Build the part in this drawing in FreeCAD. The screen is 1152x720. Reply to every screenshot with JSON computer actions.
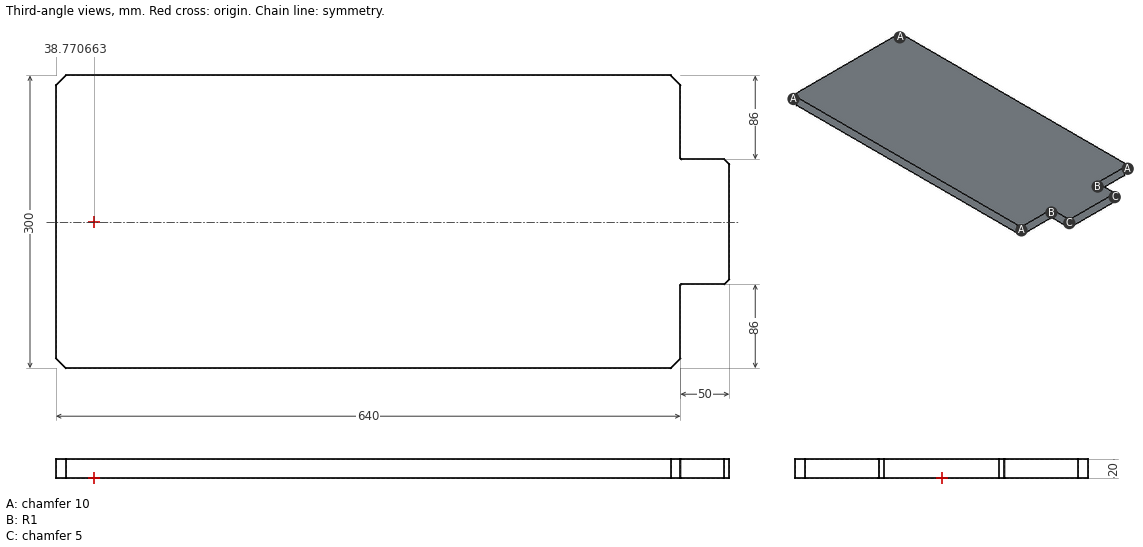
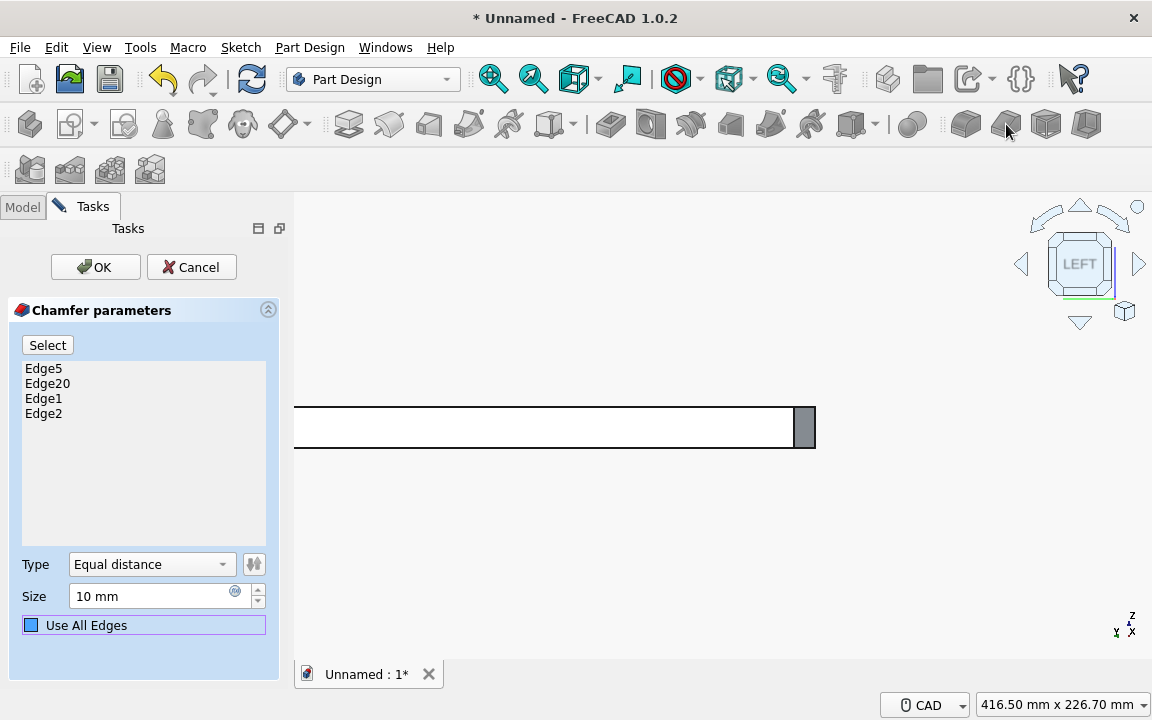
{"action": "left_click", "coordinate": [96, 267]}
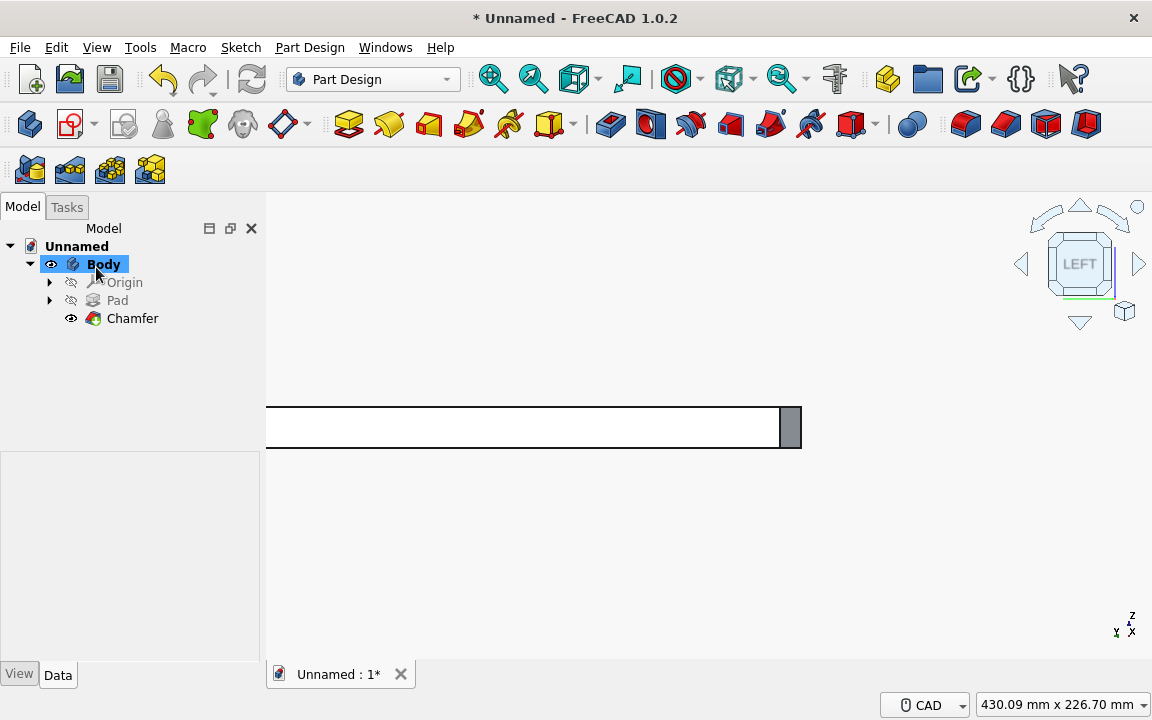
{"action": "left_click", "coordinate": [494, 80]}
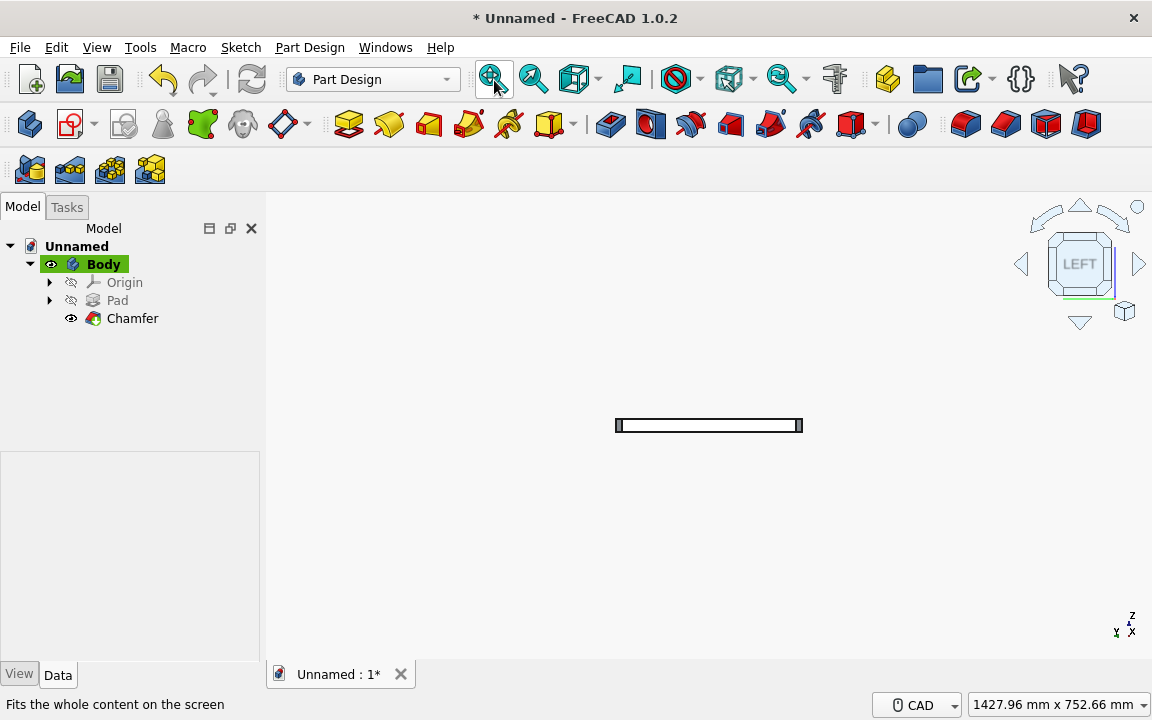
{"action": "scroll", "coordinate": [669, 424], "scroll_direction": "up", "scroll_amount": 6}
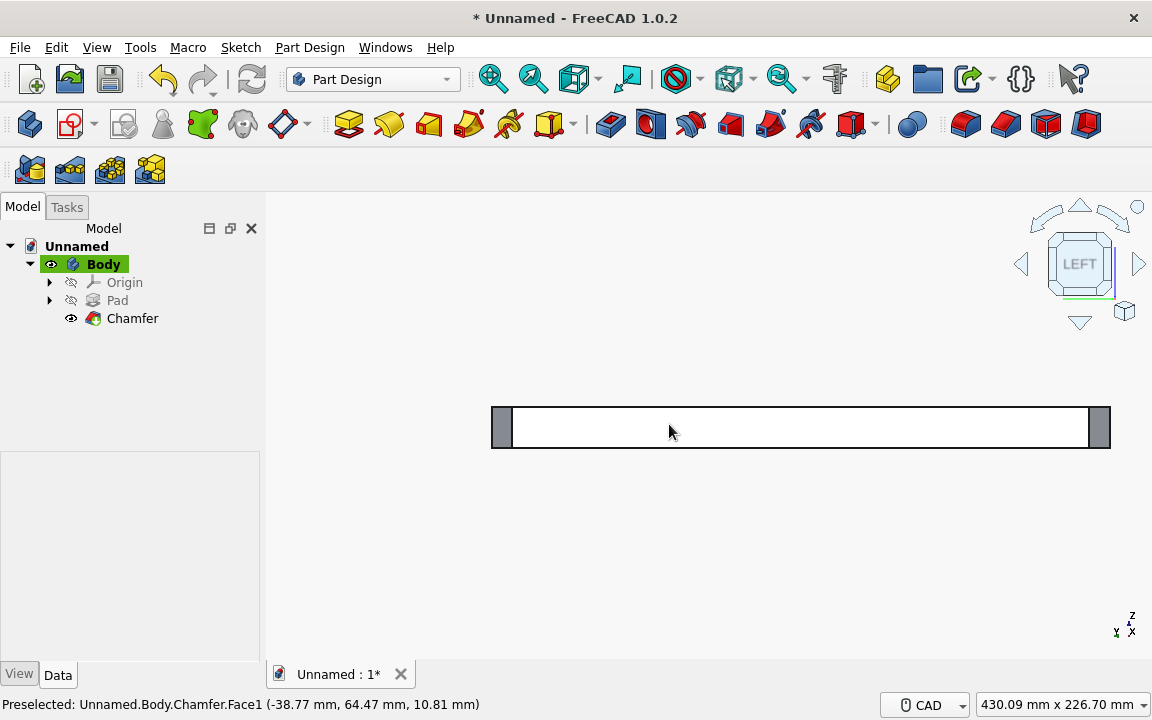
{"action": "key", "text": "v f"}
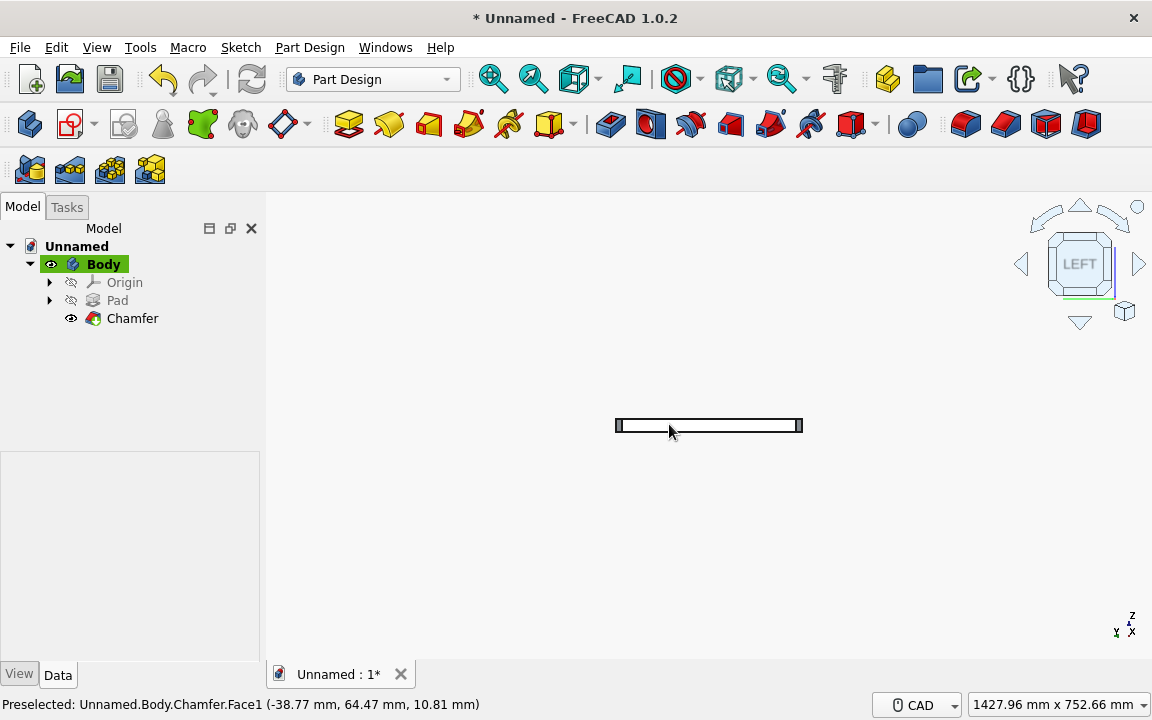
{"action": "key", "text": "0"}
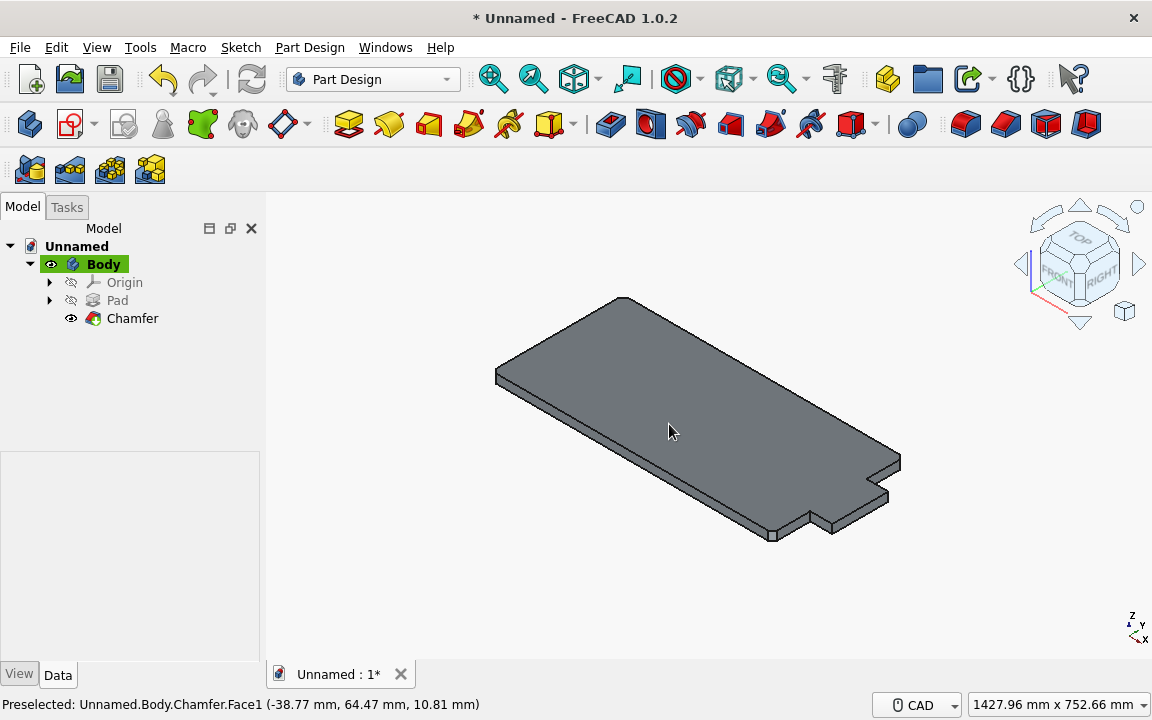
{"action": "scroll", "coordinate": [867, 483], "scroll_direction": "up", "scroll_amount": 6}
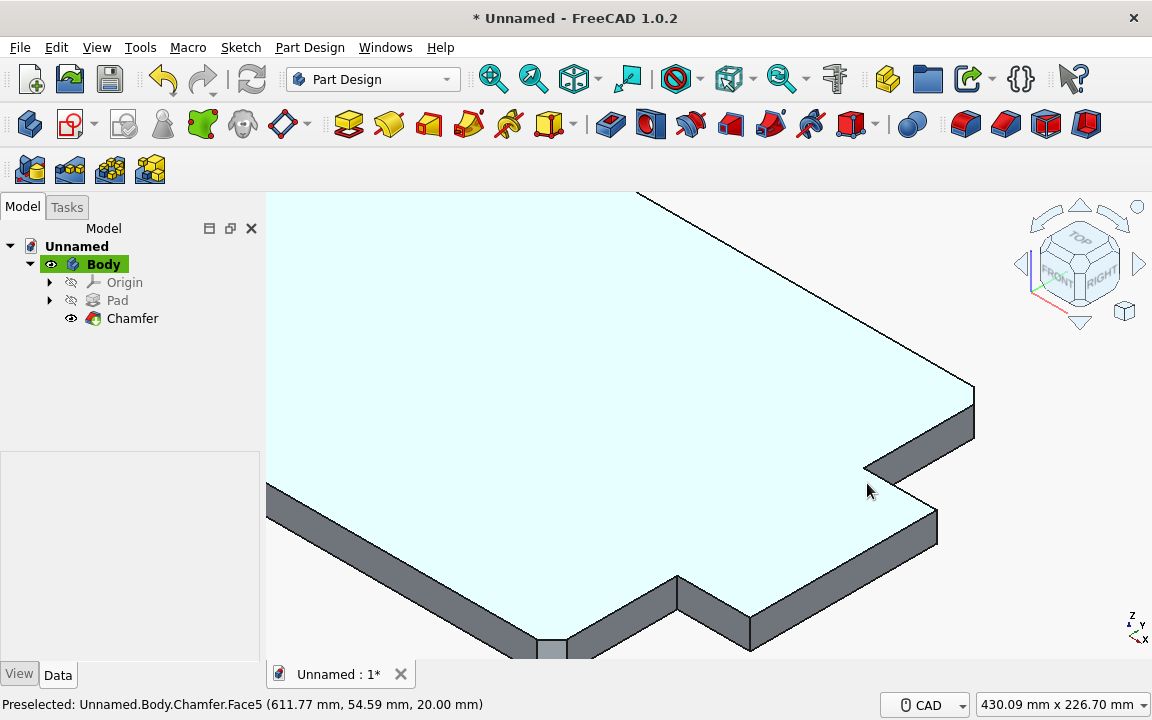
{"action": "left_click", "coordinate": [494, 80]}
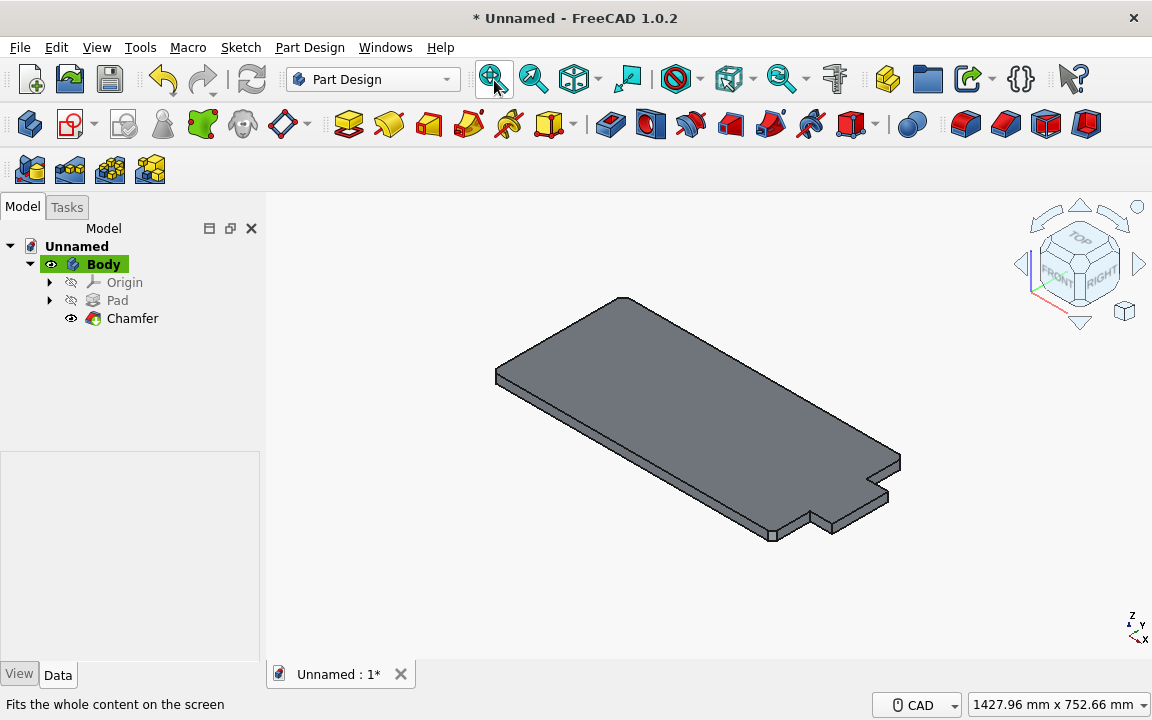
{"action": "key", "text": "2"}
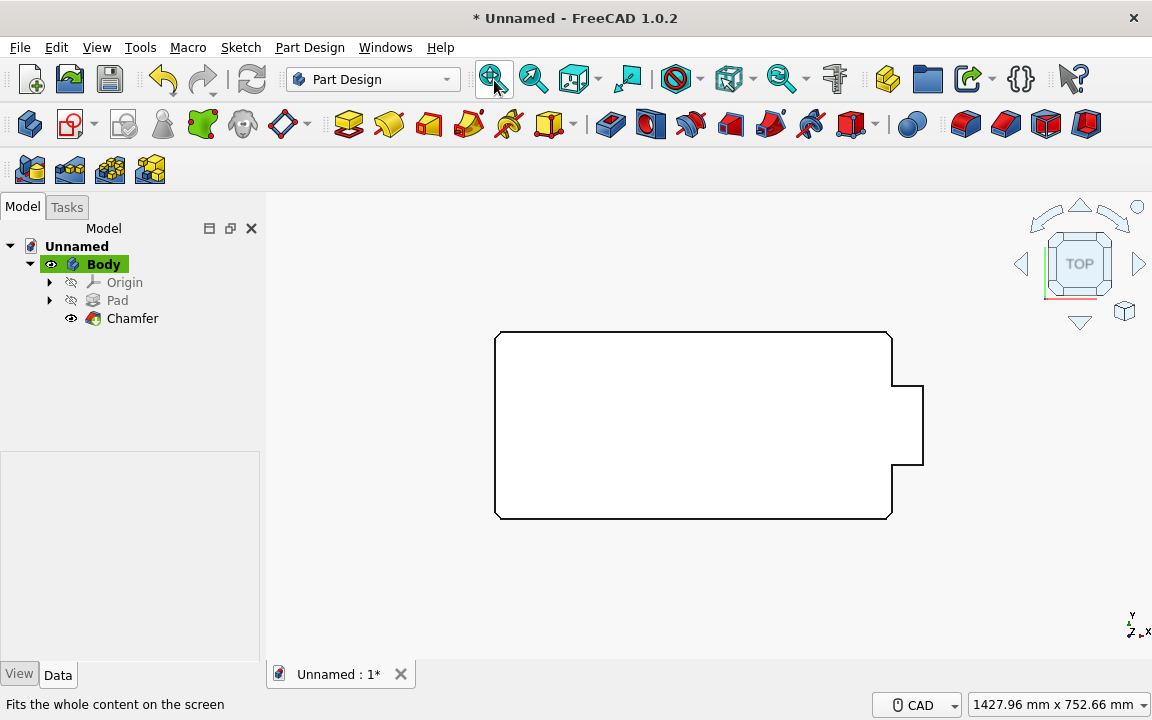
{"action": "scroll", "coordinate": [892, 385], "scroll_direction": "up", "scroll_amount": 6}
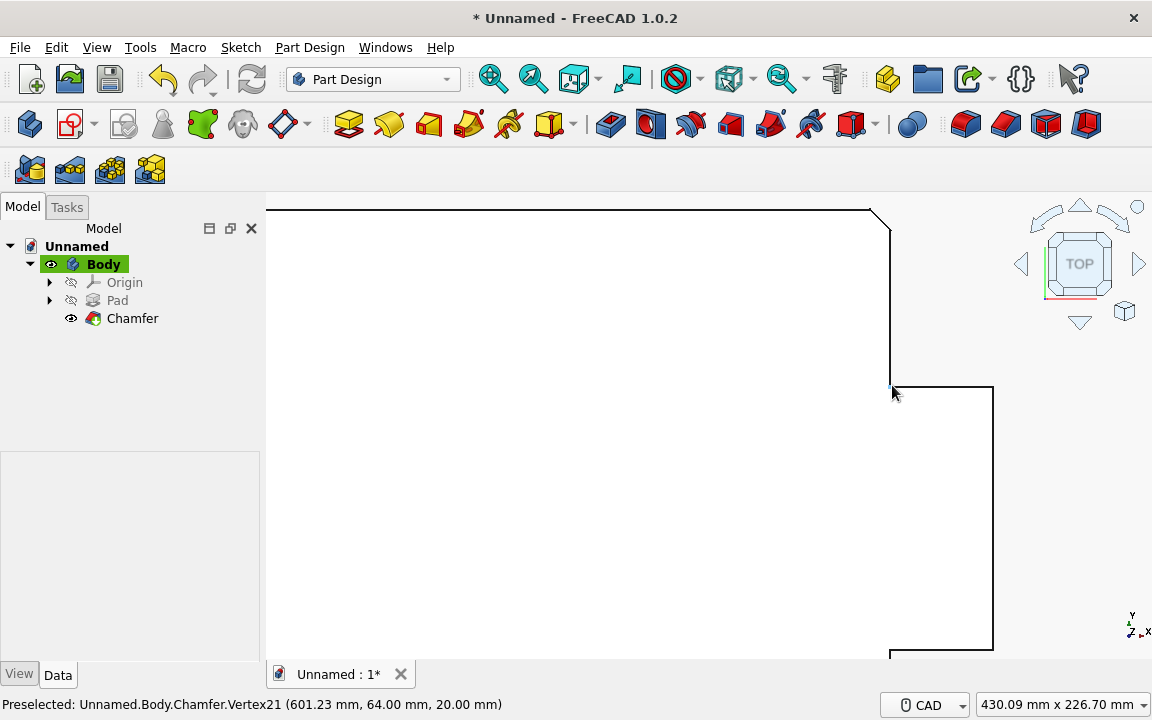
{"action": "left_click", "coordinate": [494, 80]}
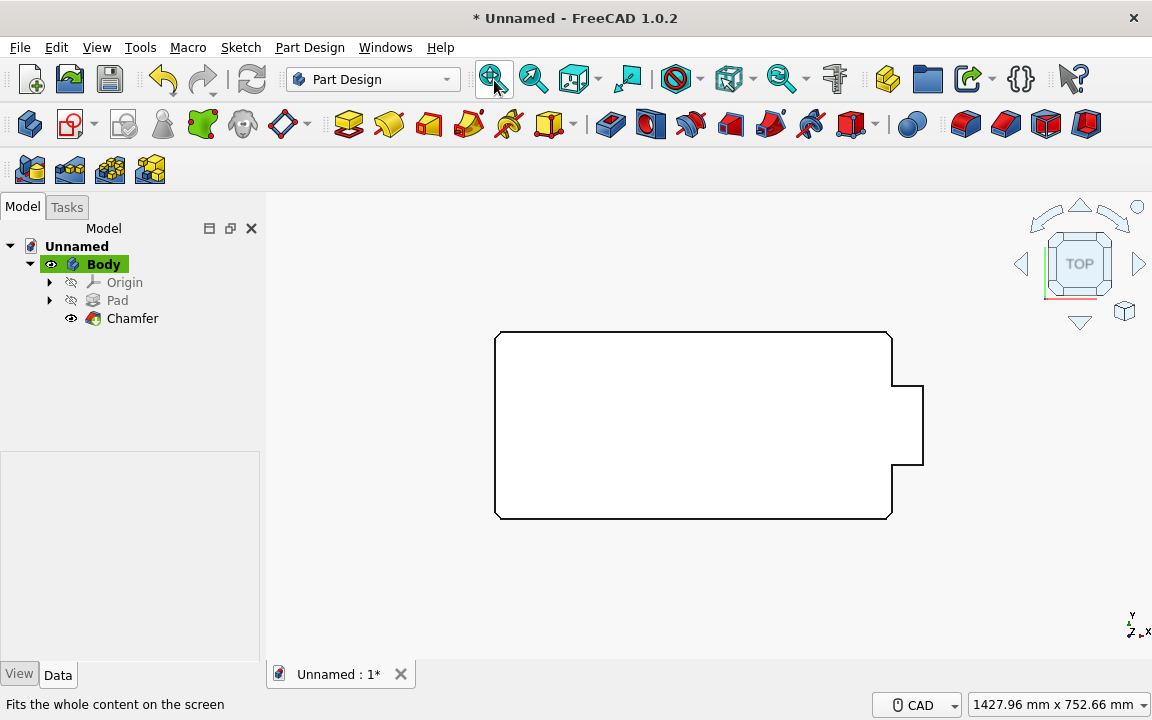
{"action": "key", "text": "1"}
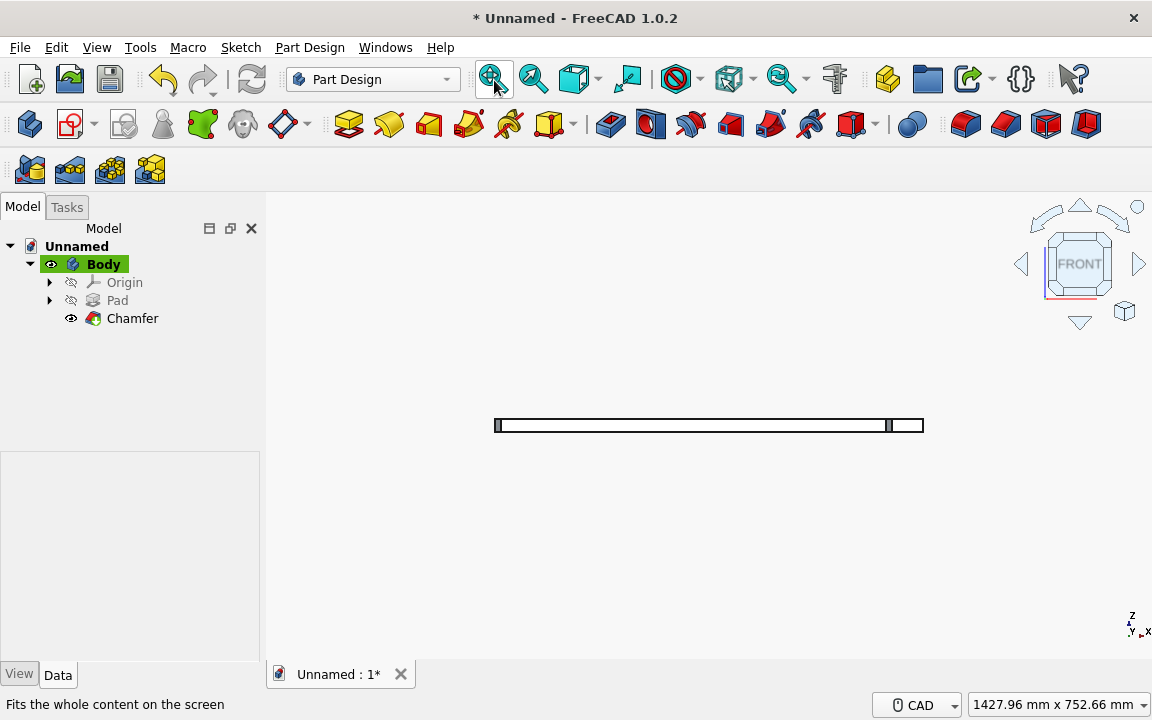
{"action": "scroll", "coordinate": [892, 424], "scroll_direction": "up", "scroll_amount": 6}